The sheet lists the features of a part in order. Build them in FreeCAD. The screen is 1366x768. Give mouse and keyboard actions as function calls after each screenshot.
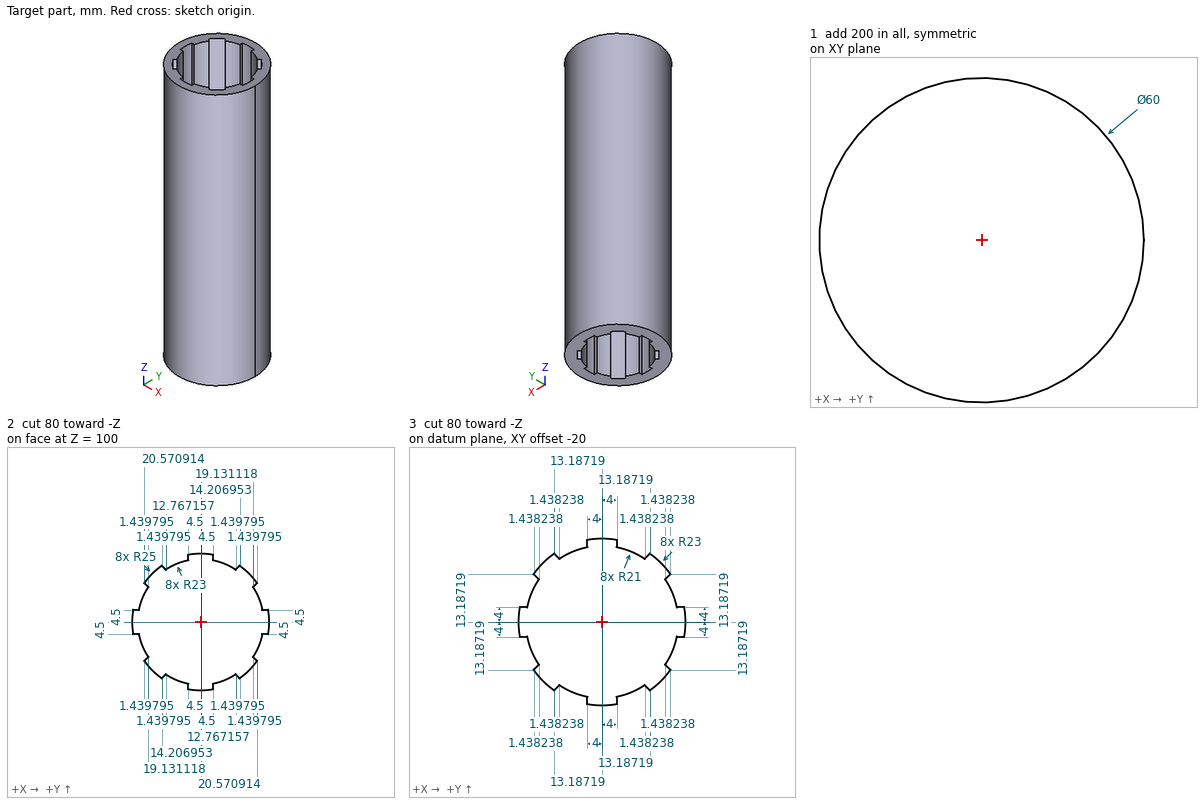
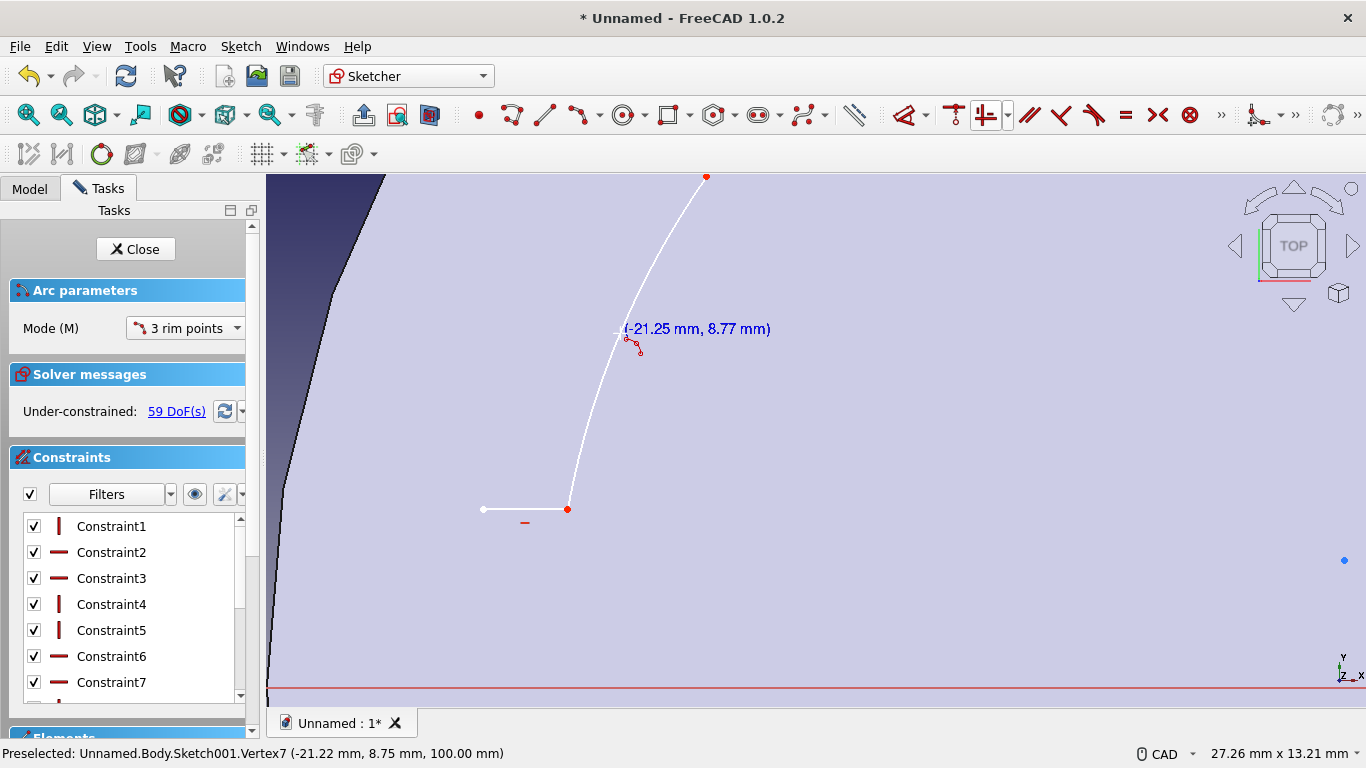
click(483, 509)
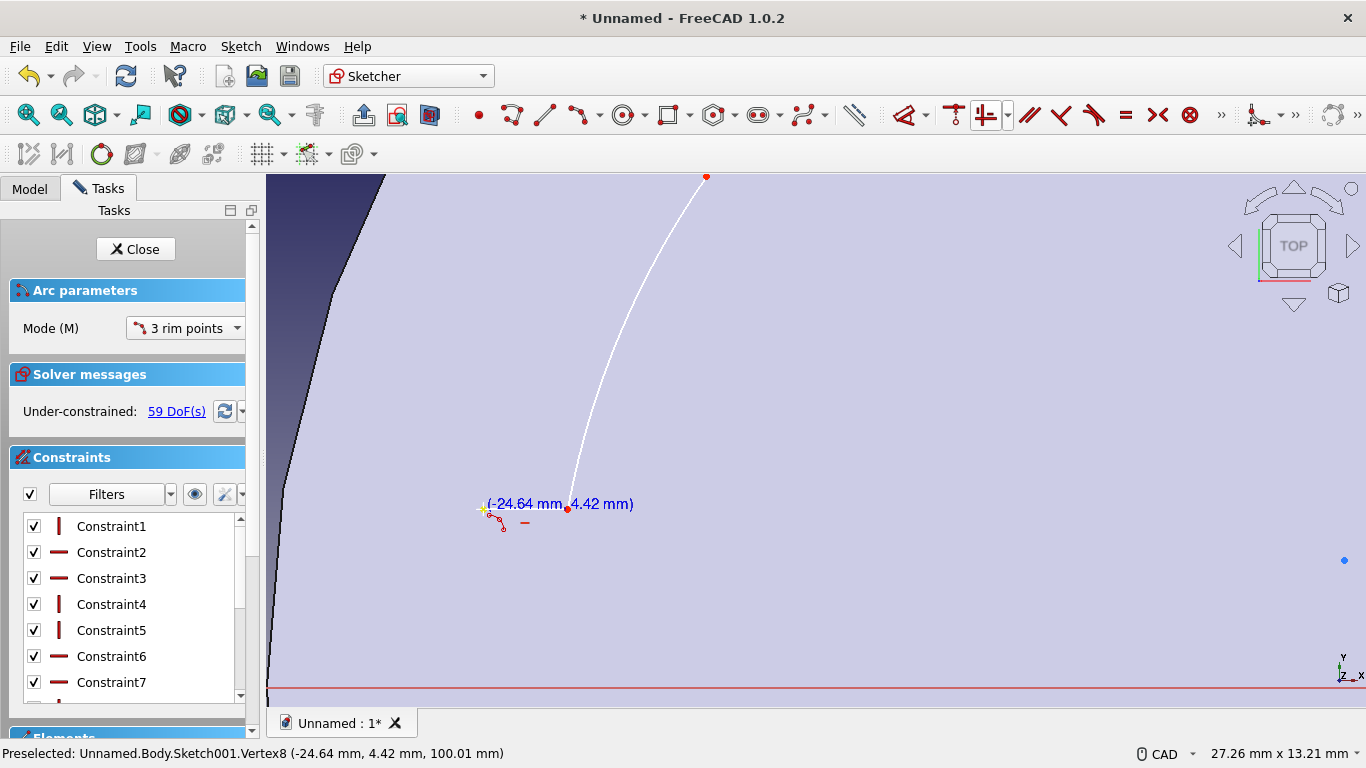
scroll(603, 392, down, 9)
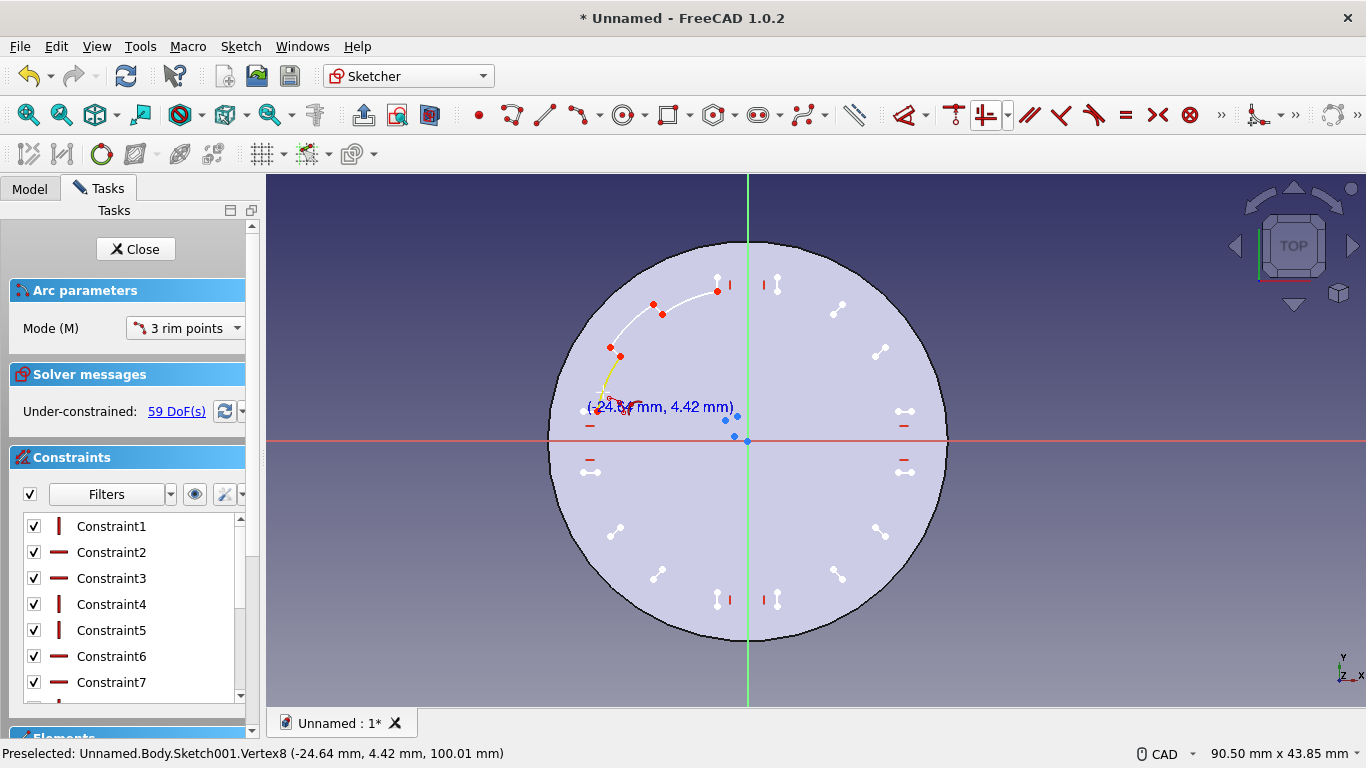
scroll(584, 471, up, 5)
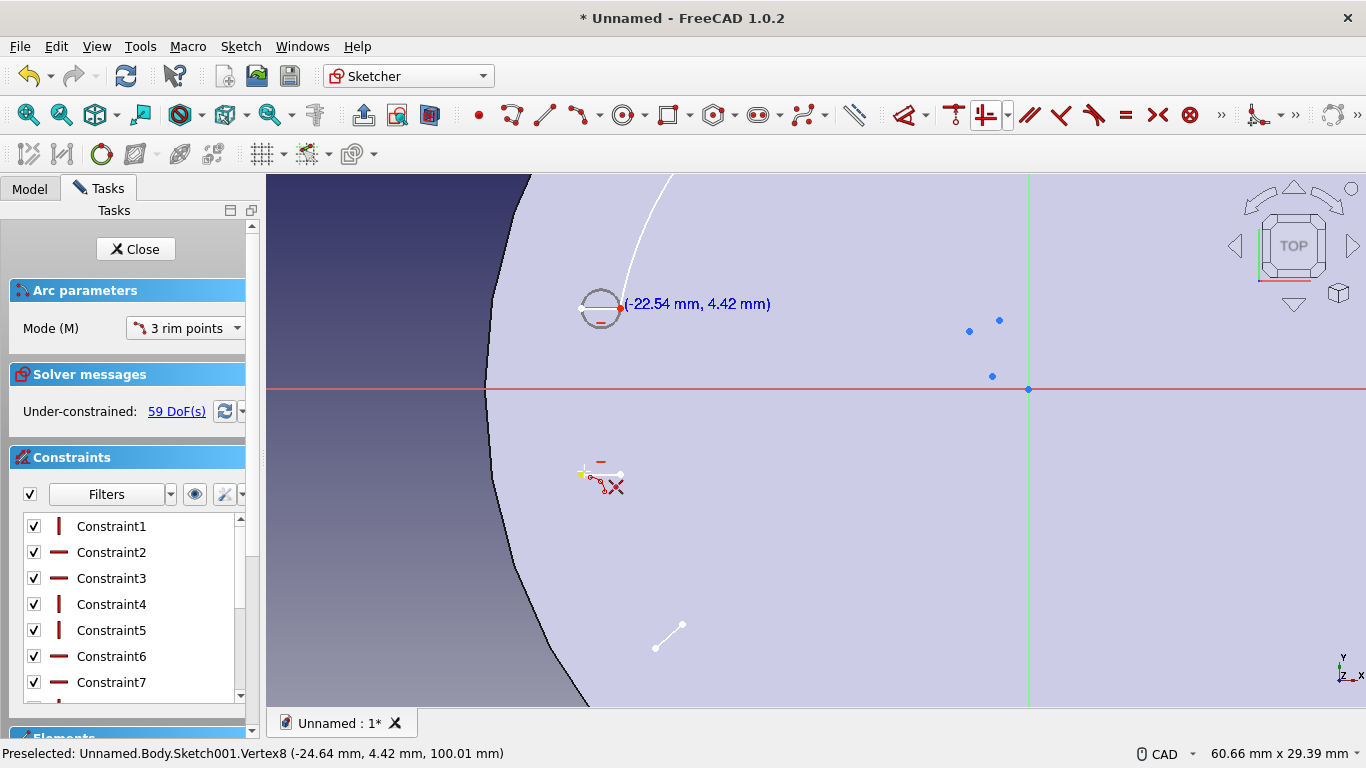
click(582, 475)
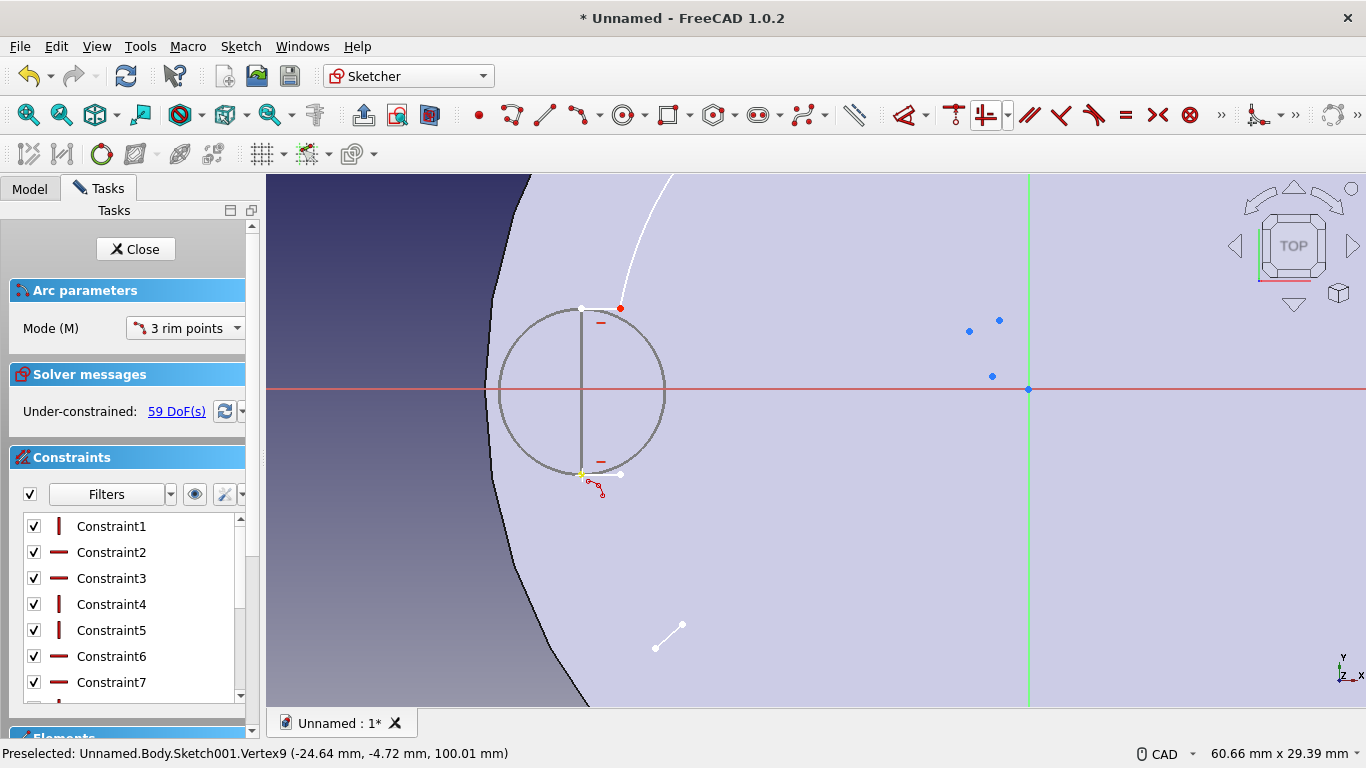
scroll(576, 373, up, 5)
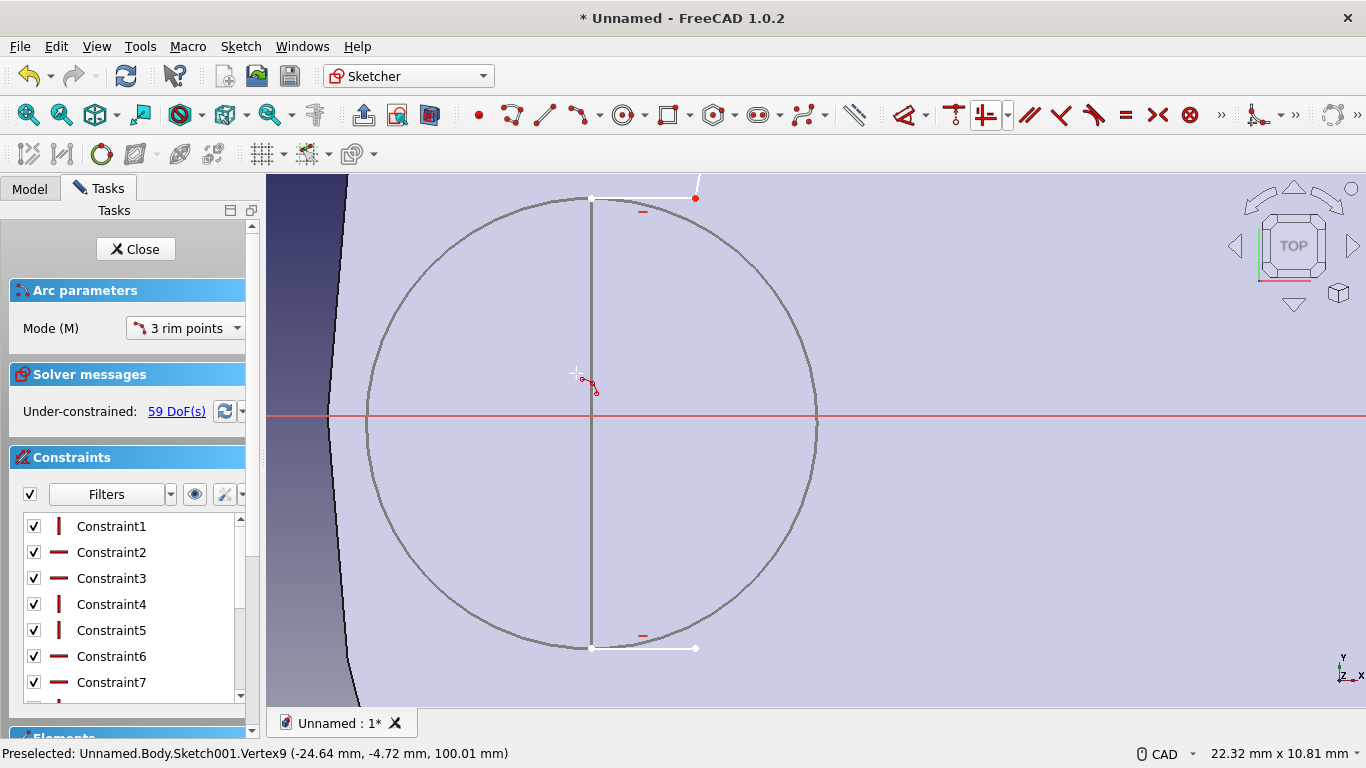
click(575, 372)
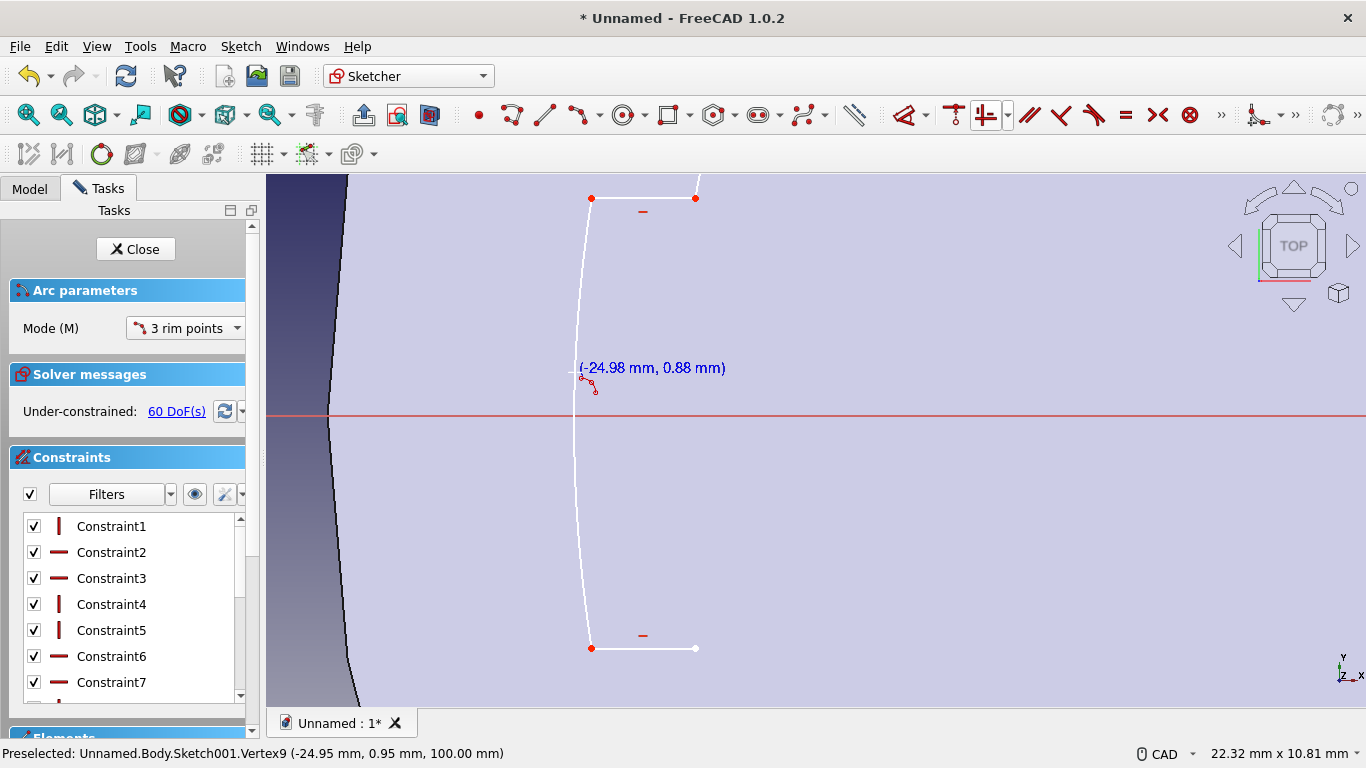
scroll(582, 444, down, 10)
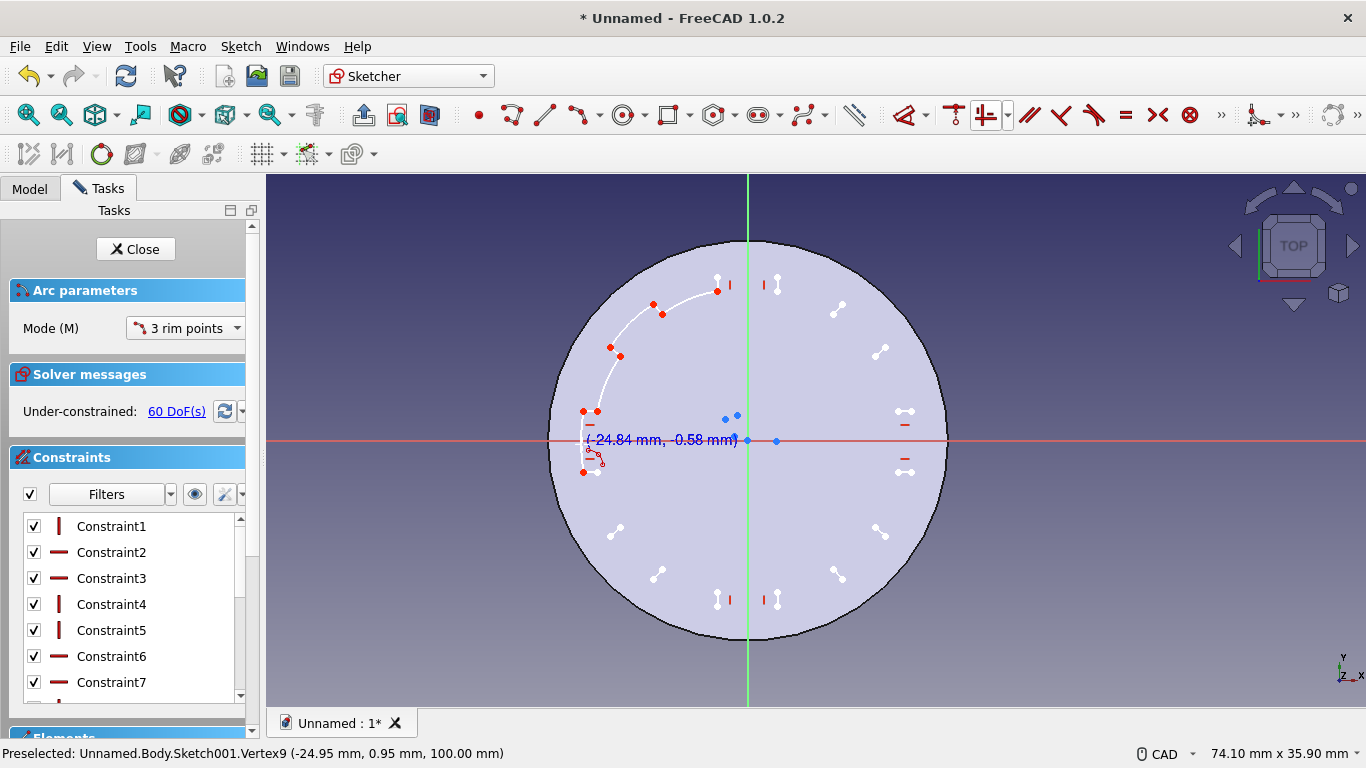
scroll(597, 471, up, 5)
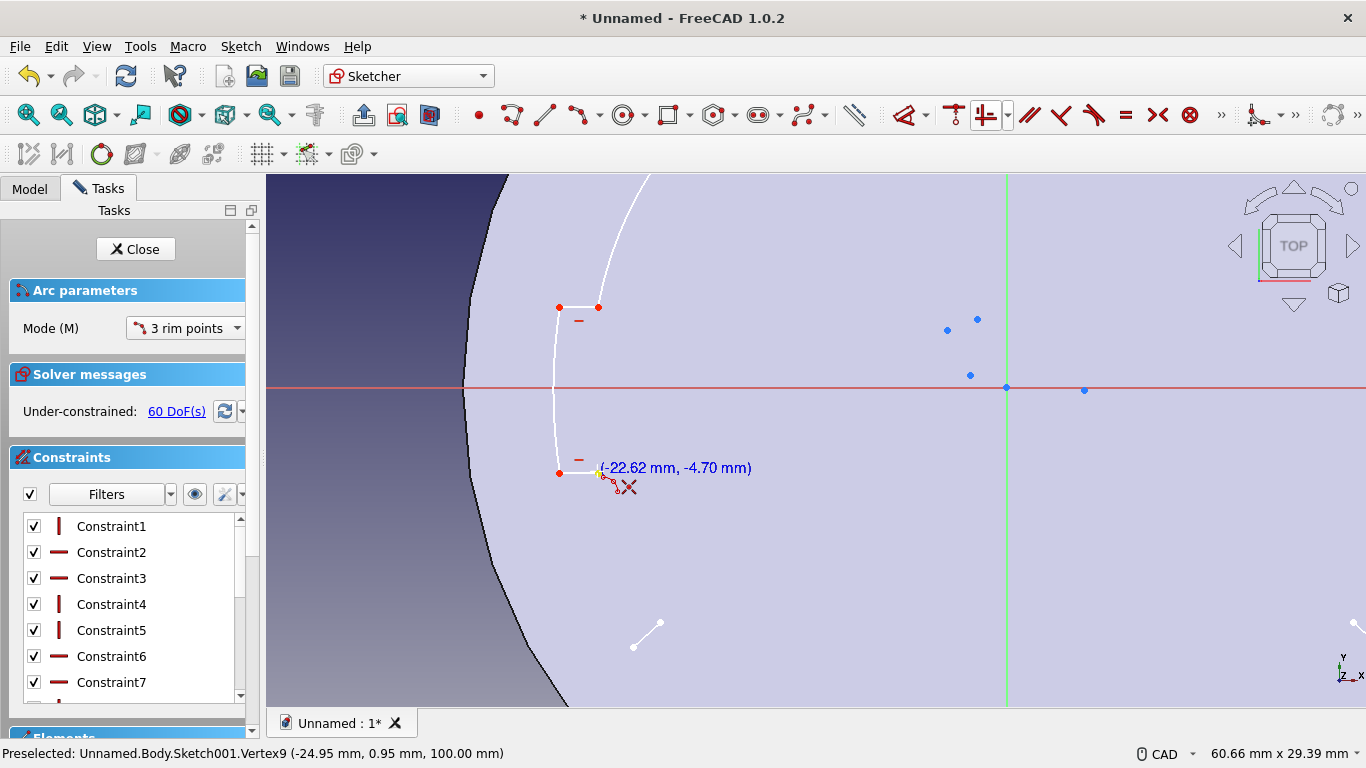
click(598, 473)
click(661, 623)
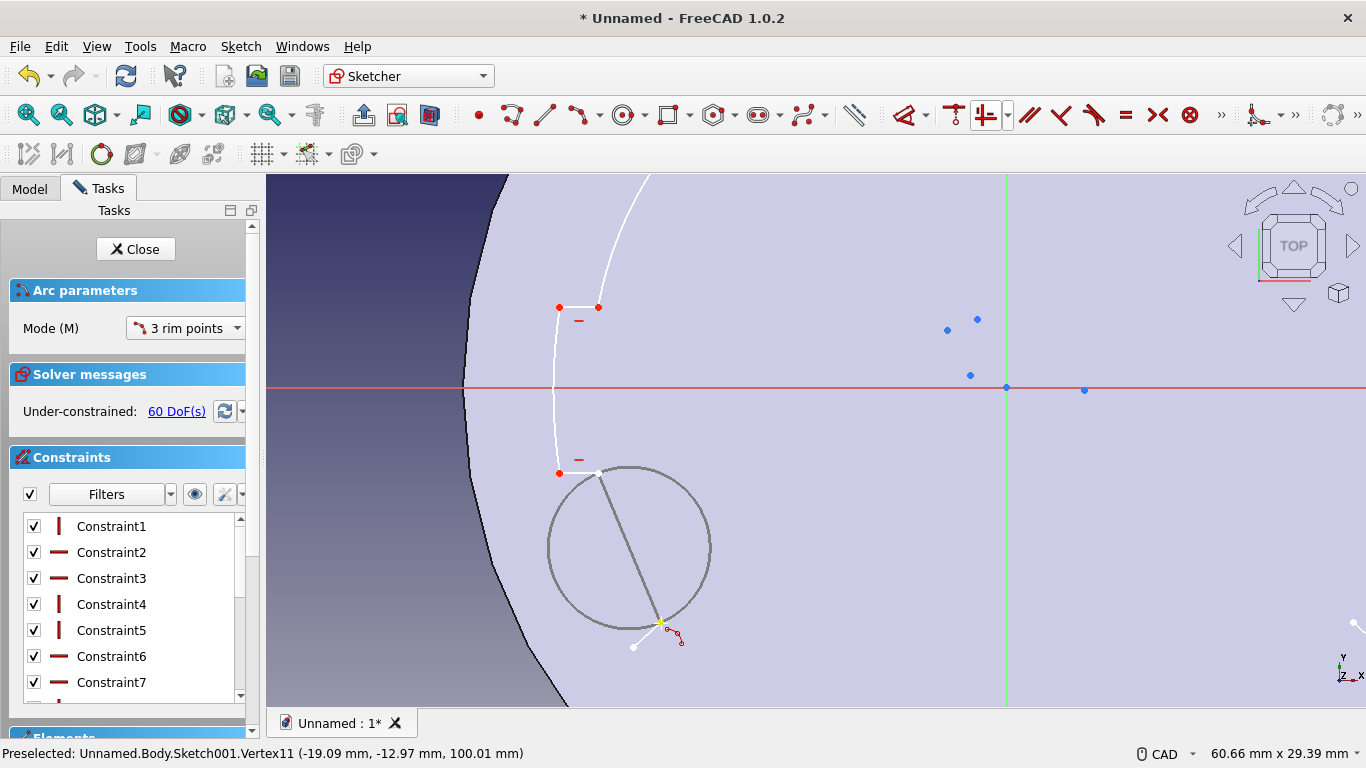
scroll(621, 547, up, 4)